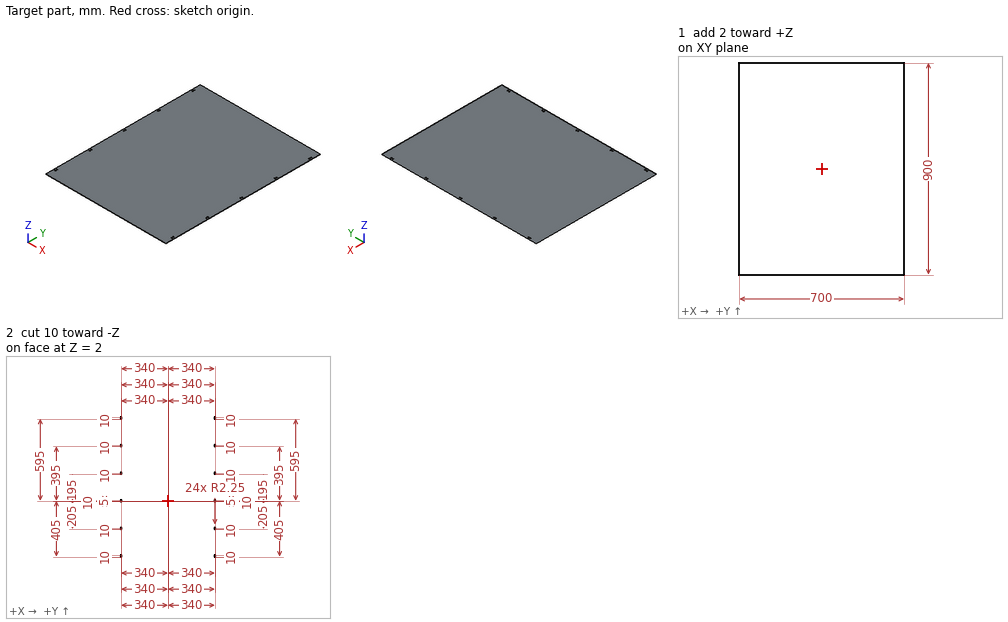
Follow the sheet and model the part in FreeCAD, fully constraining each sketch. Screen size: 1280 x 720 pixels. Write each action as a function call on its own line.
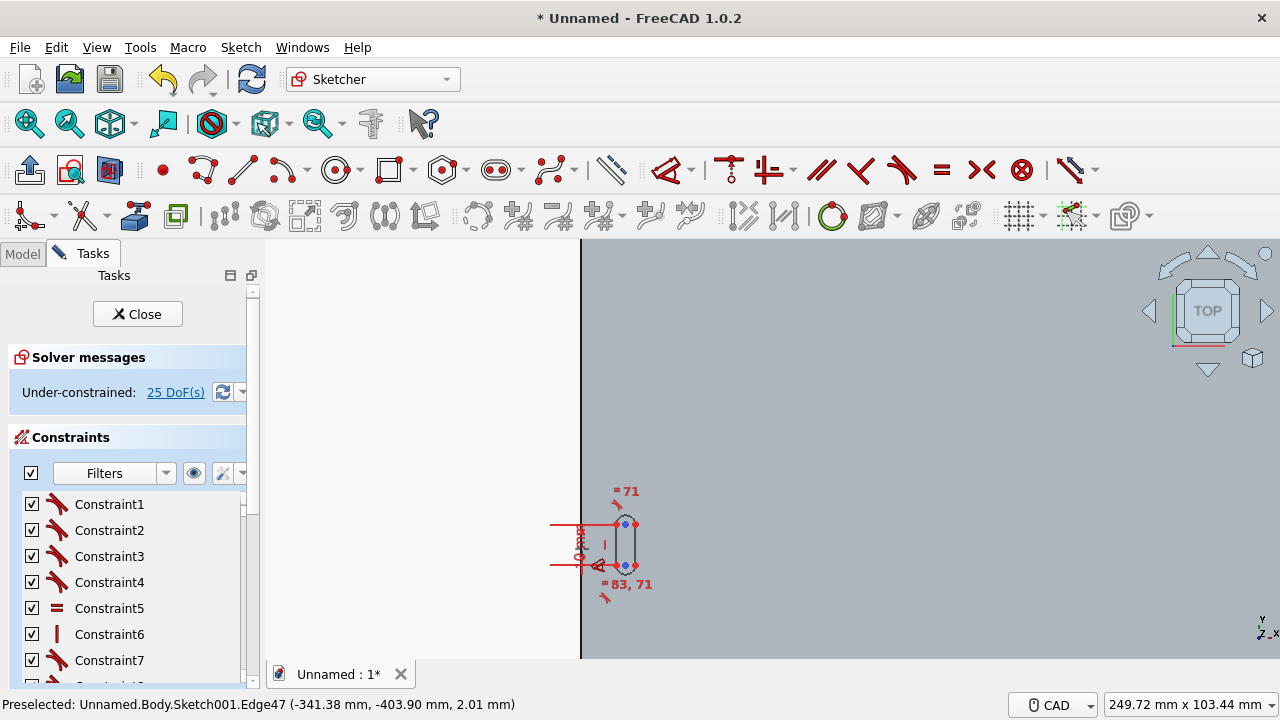
scroll(620, 574, down, 14)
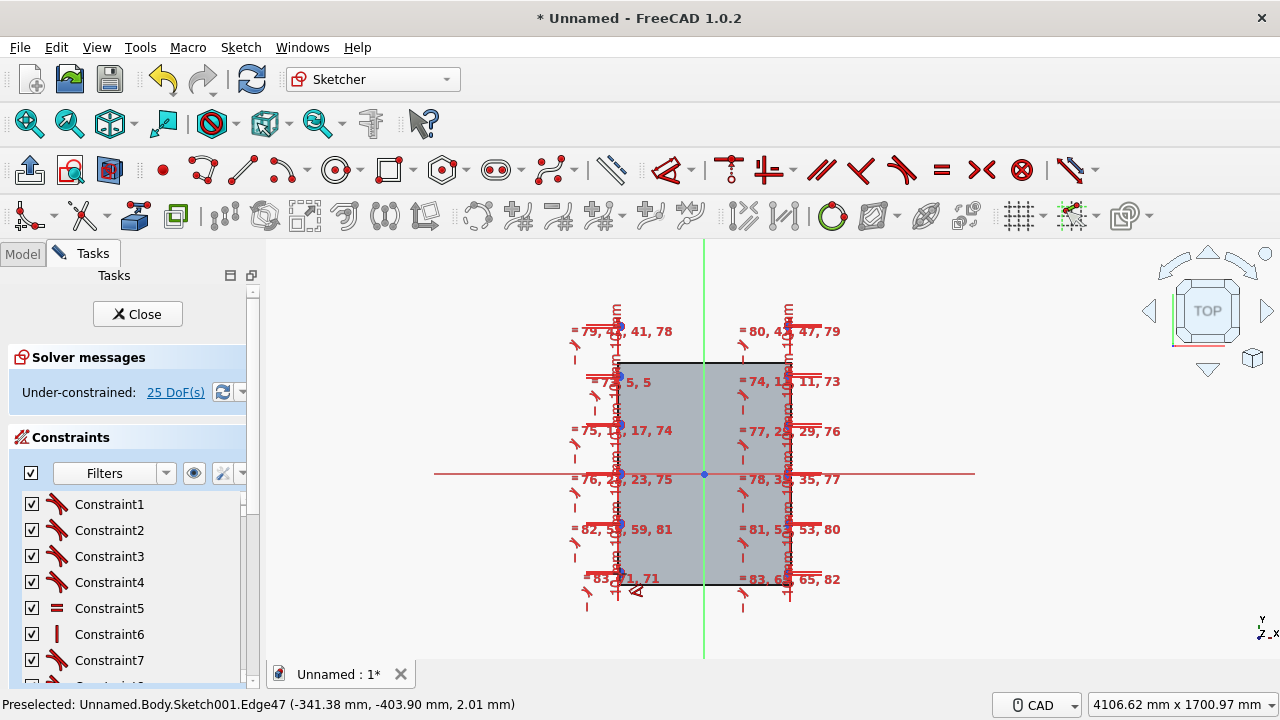
scroll(620, 475, up, 18)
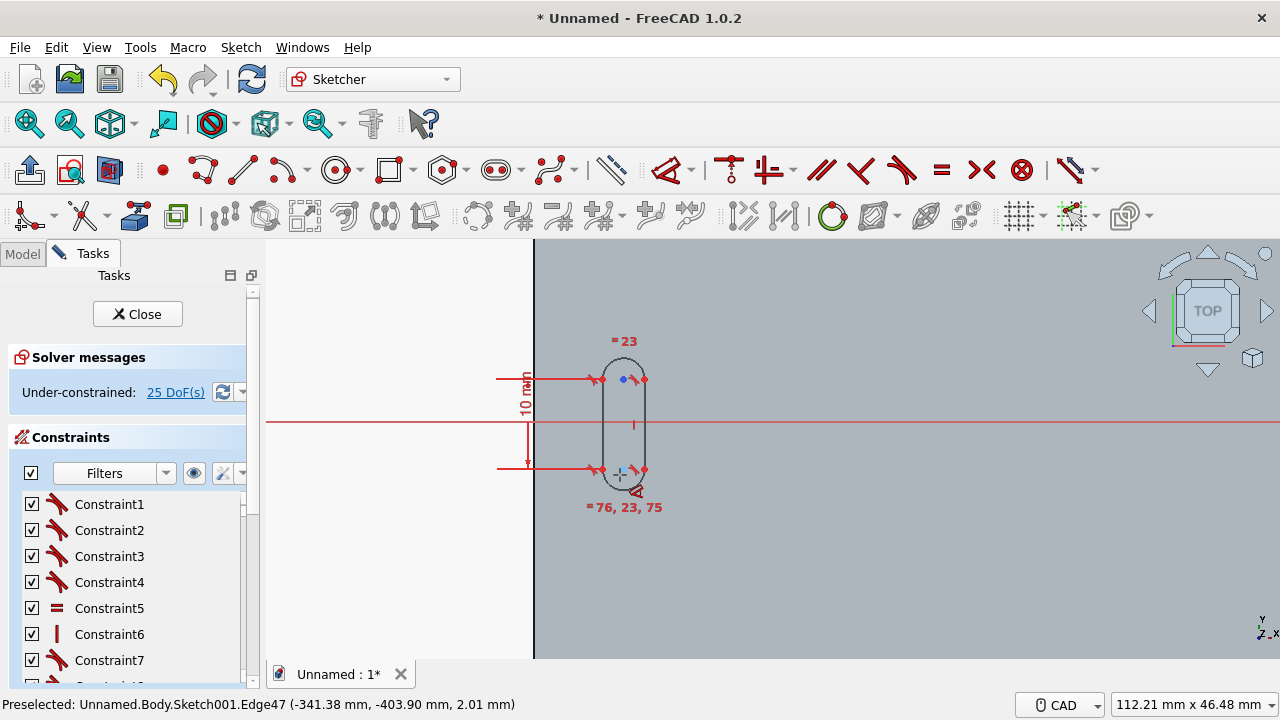
click(603, 469)
click(569, 446)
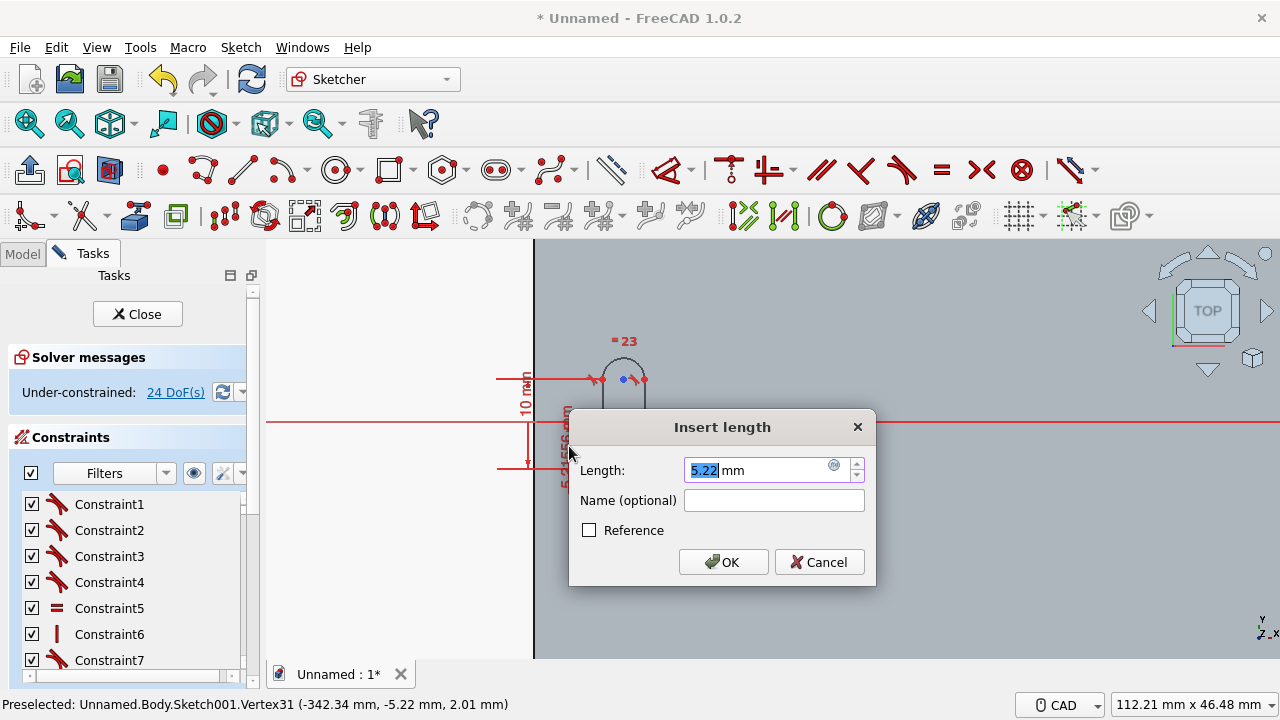
text(5)
key(Return)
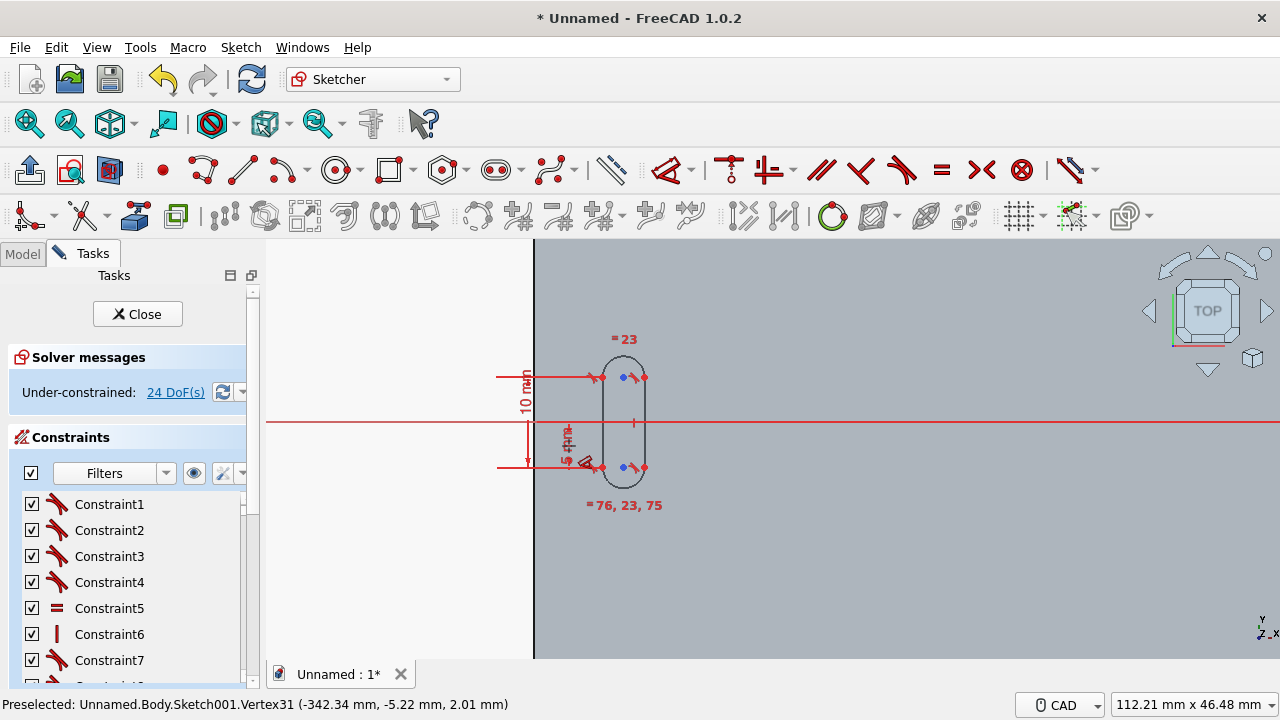
scroll(601, 481, down, 17)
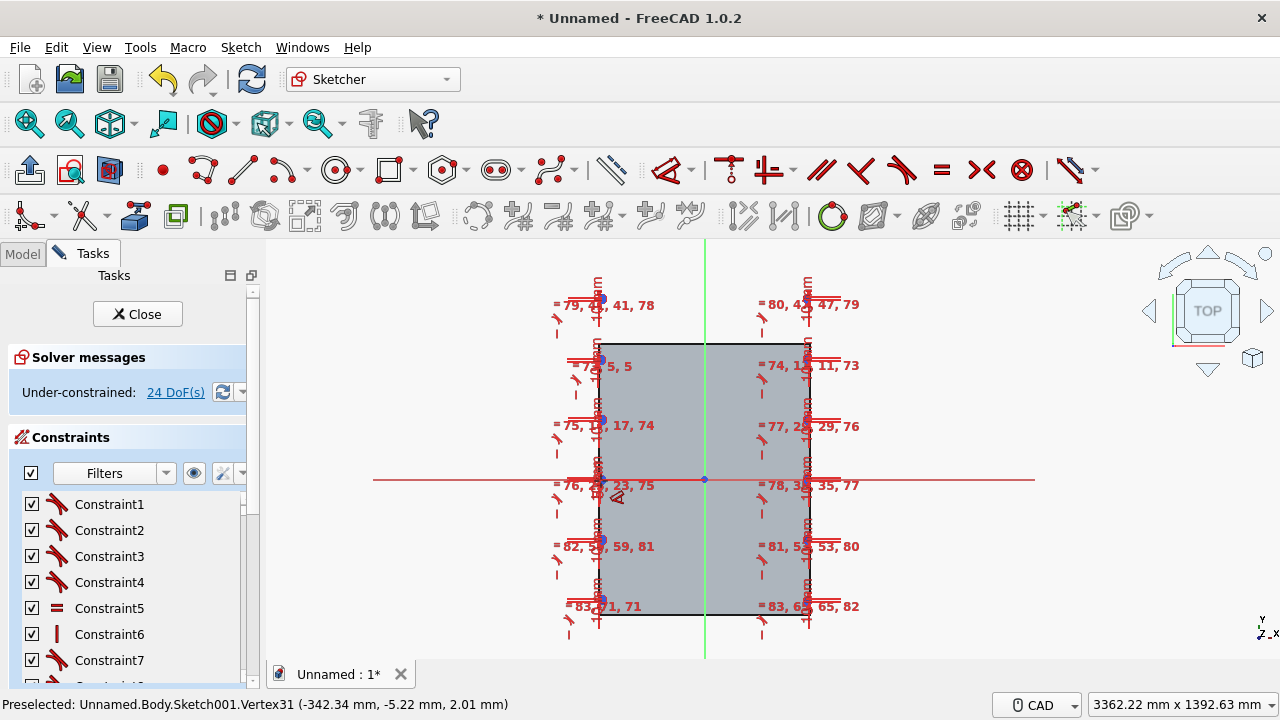
scroll(806, 481, up, 17)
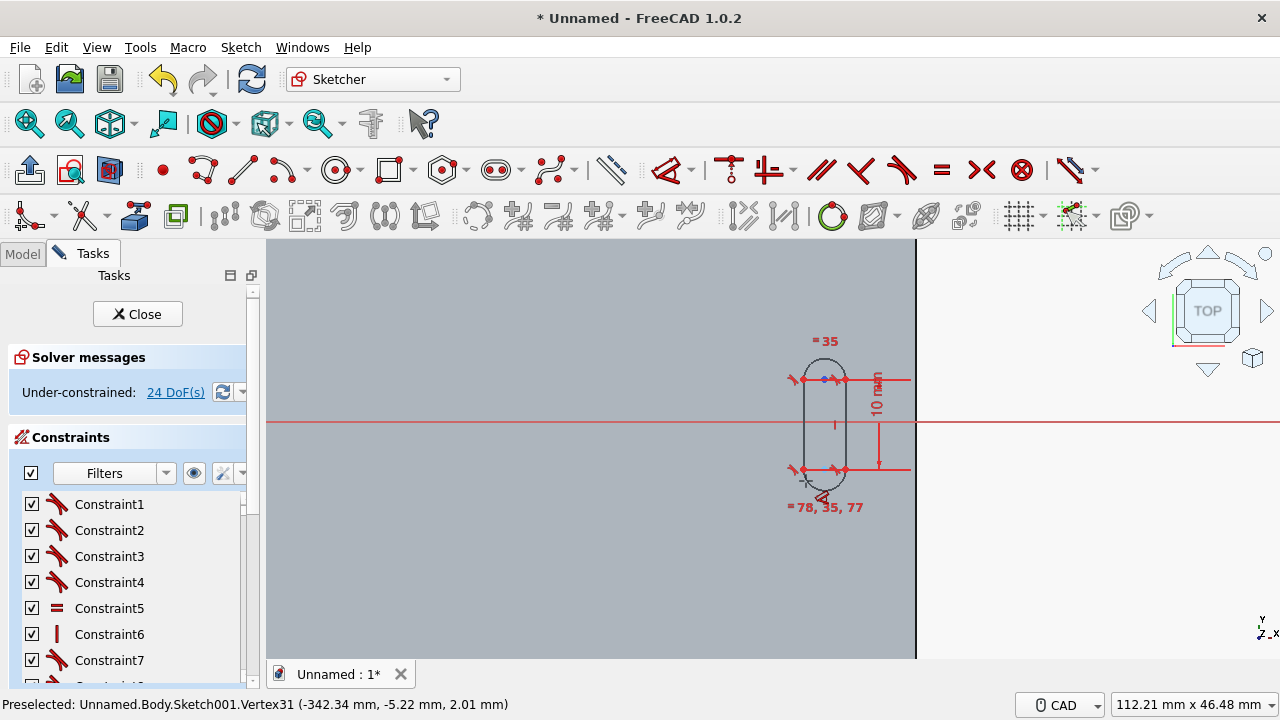
click(804, 470)
click(862, 446)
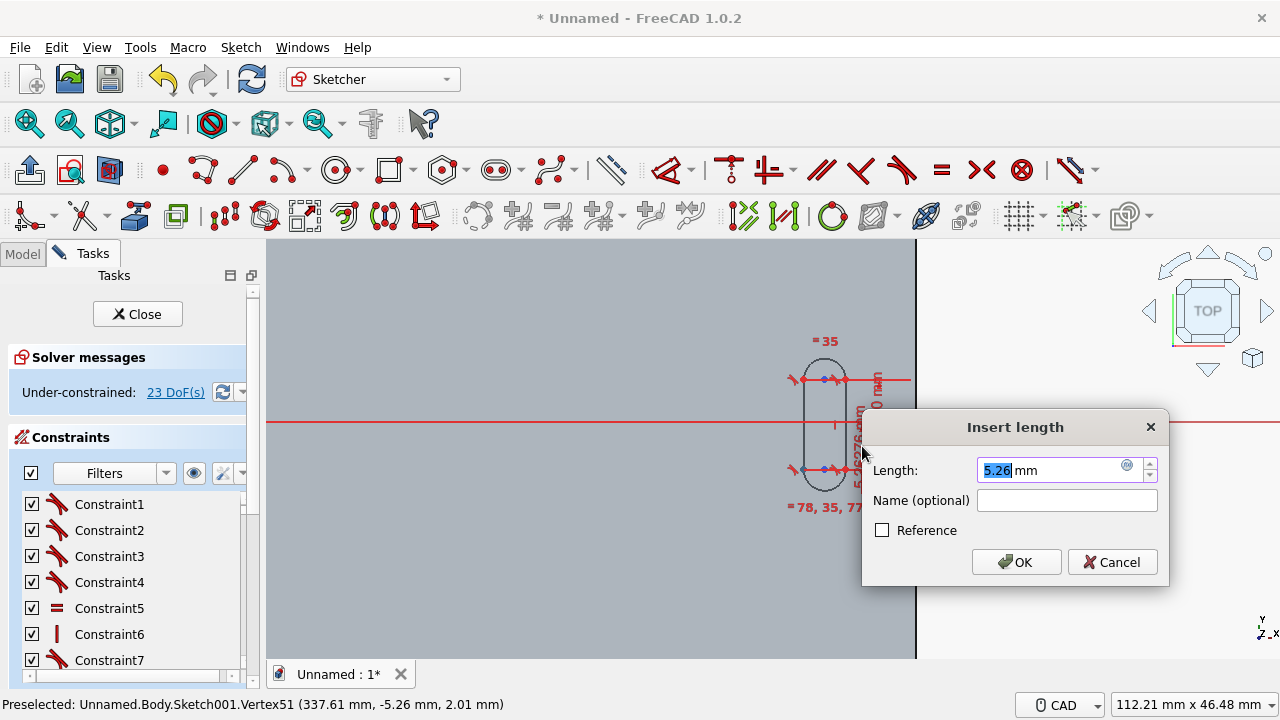
text(5)
key(Return)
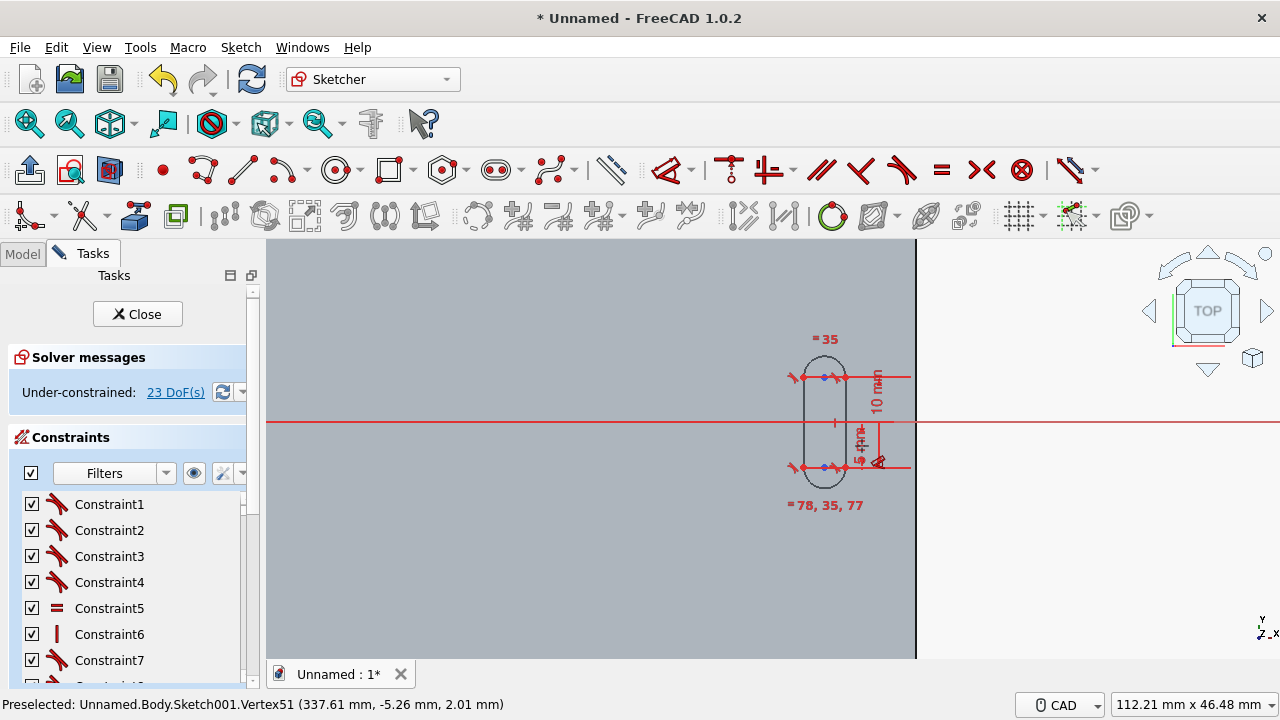
scroll(806, 481, down, 17)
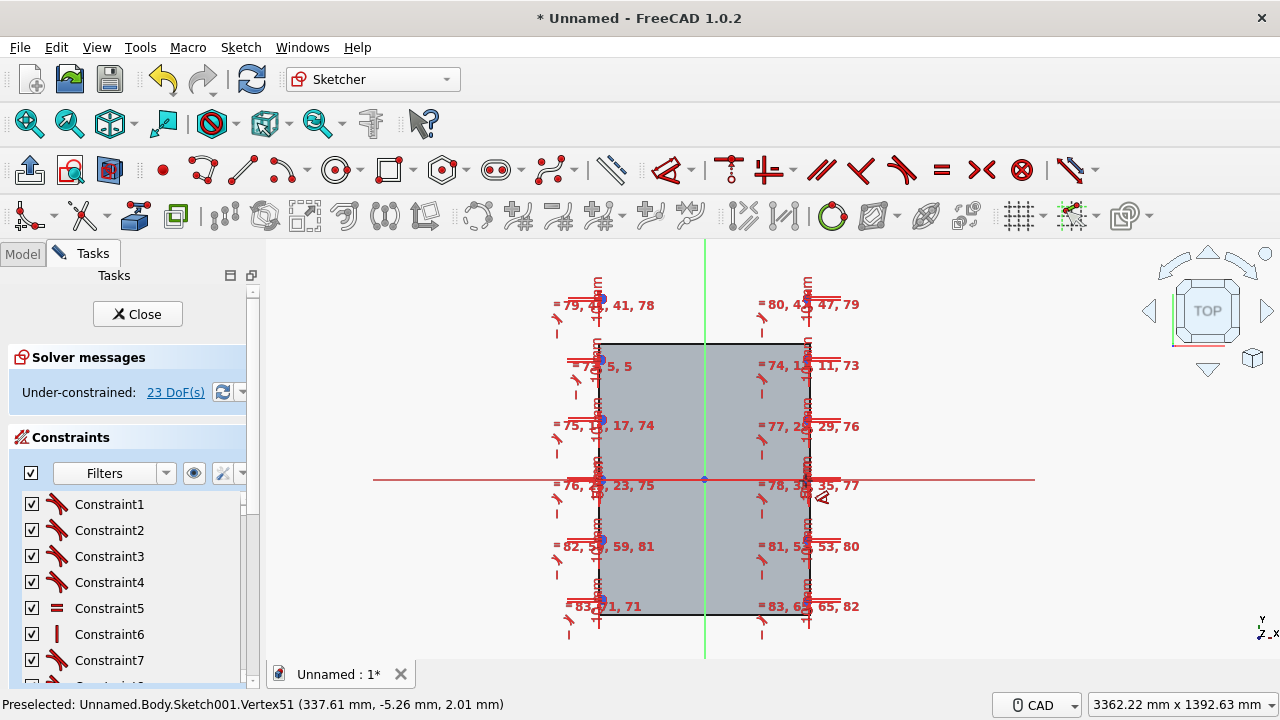
scroll(601, 362, up, 13)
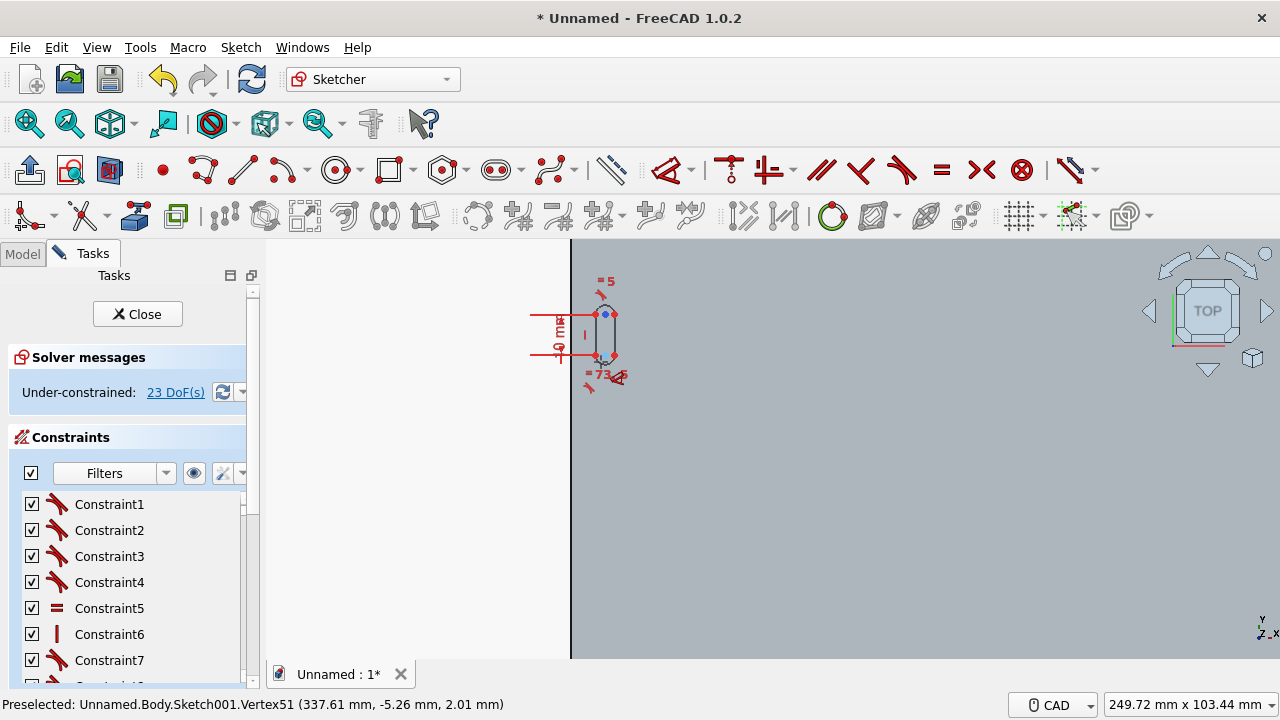
click(596, 355)
click(562, 493)